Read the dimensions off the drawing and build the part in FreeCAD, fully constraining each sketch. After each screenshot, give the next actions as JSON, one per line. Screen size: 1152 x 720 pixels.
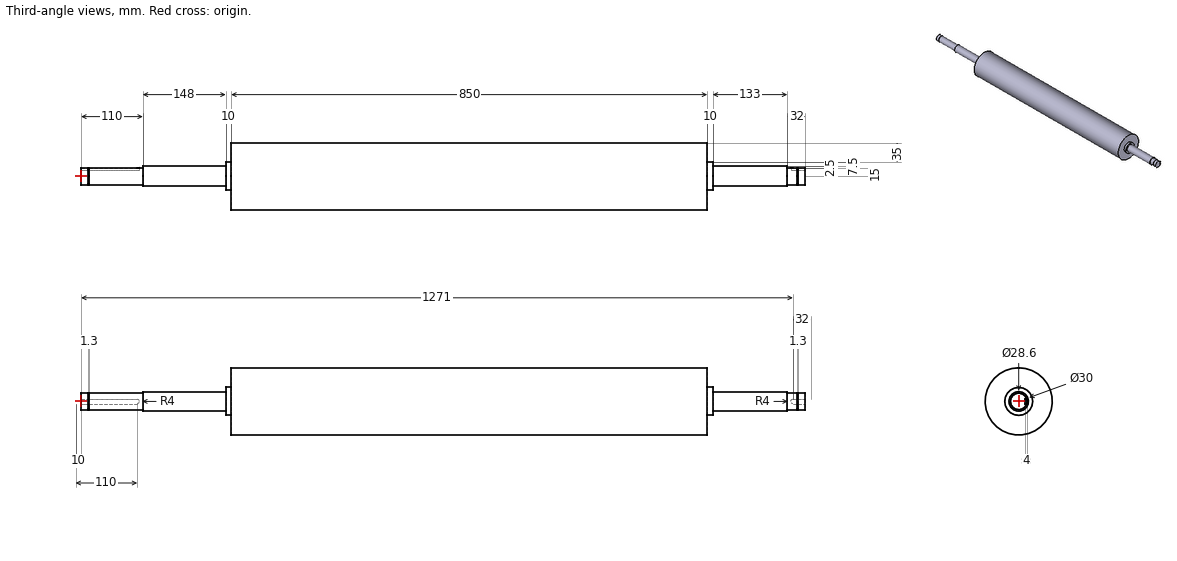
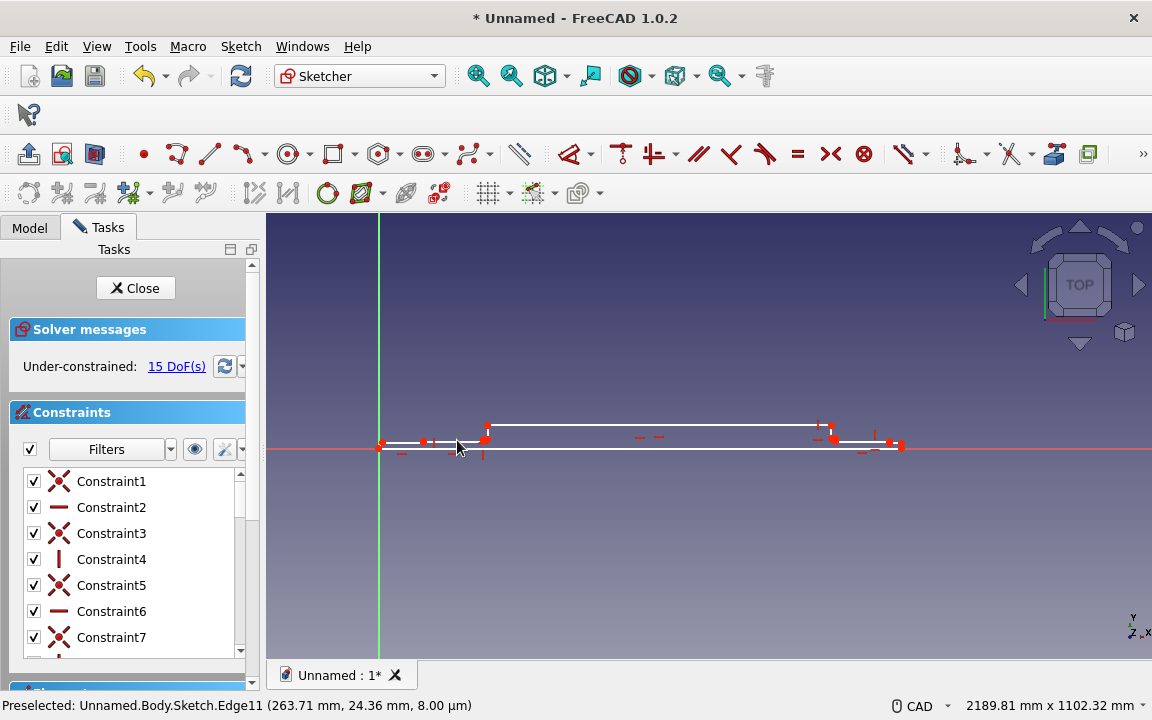
{"action": "scroll", "coordinate": [381, 445], "scroll_direction": "up", "scroll_amount": 10}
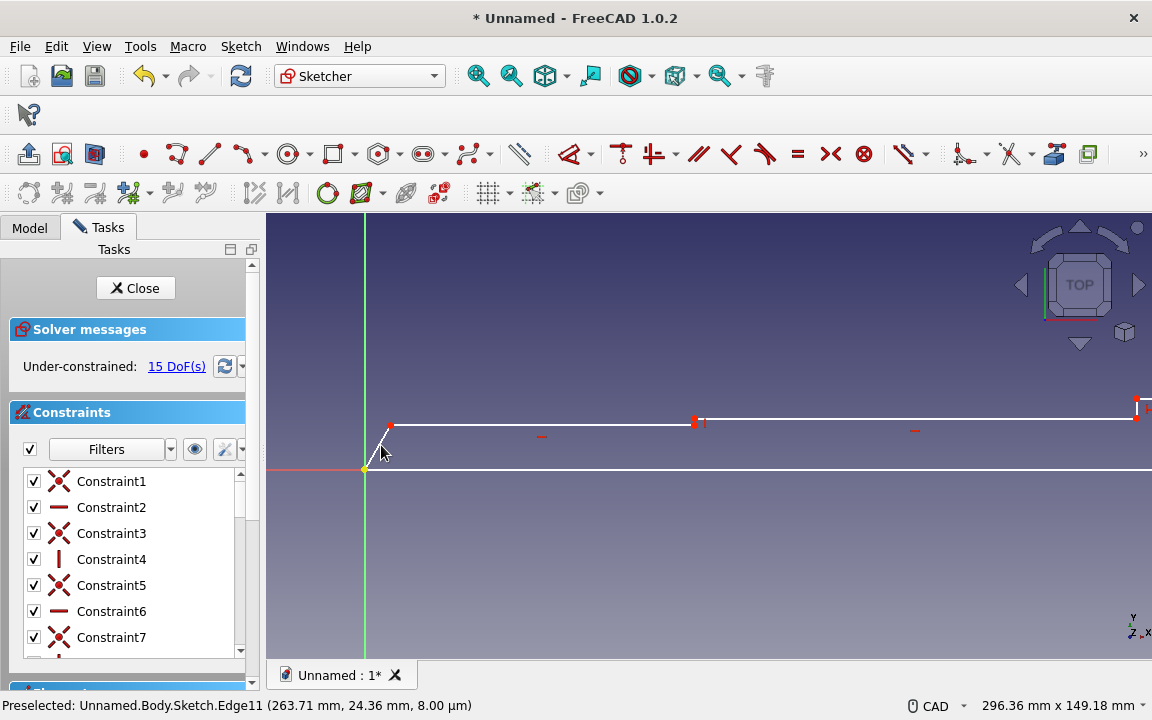
{"action": "left_click", "coordinate": [383, 439]}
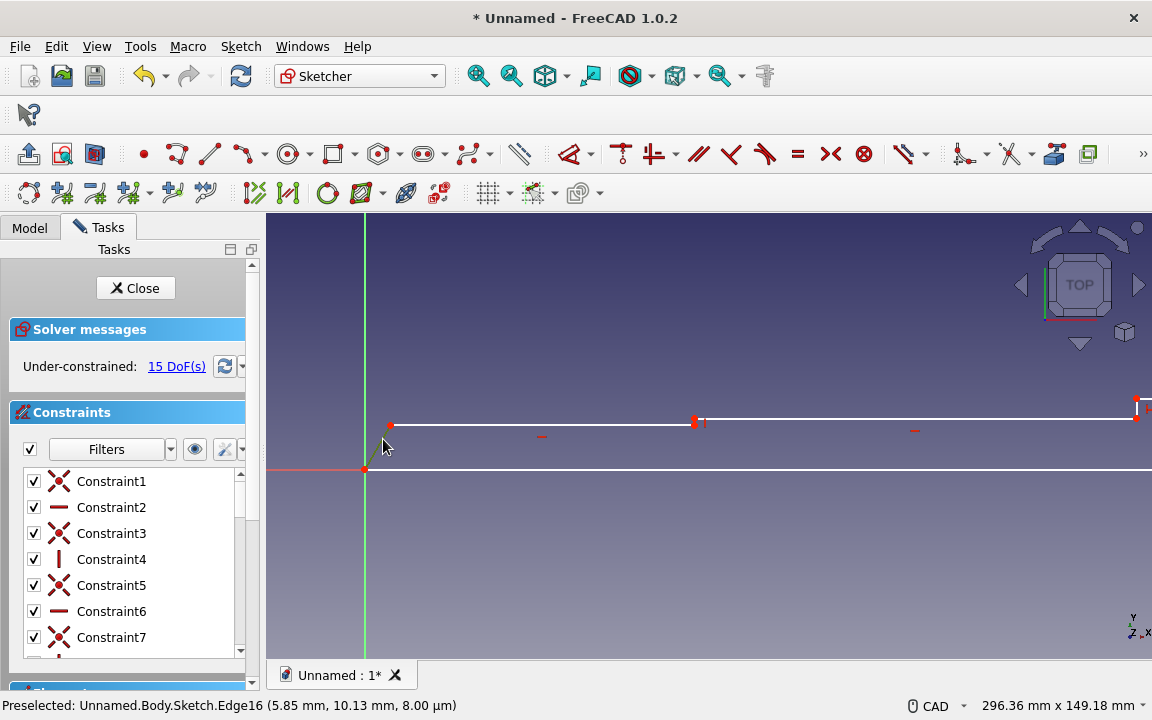
{"action": "left_click", "coordinate": [676, 154]}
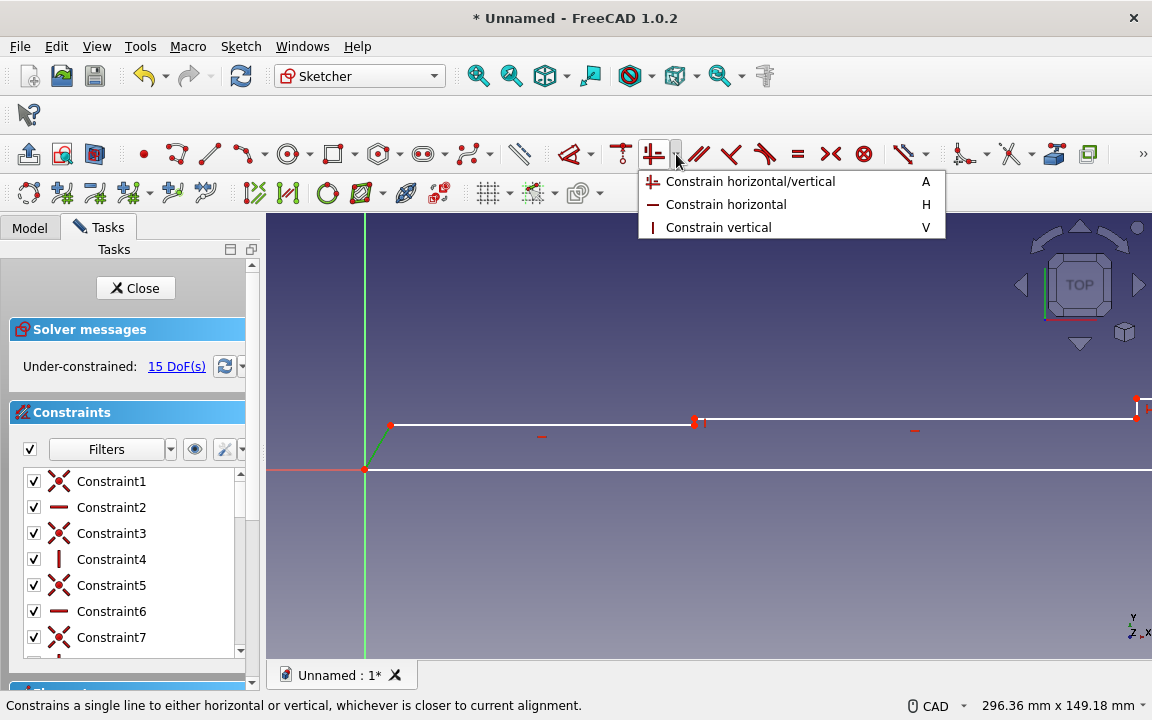
{"action": "left_click", "coordinate": [792, 228]}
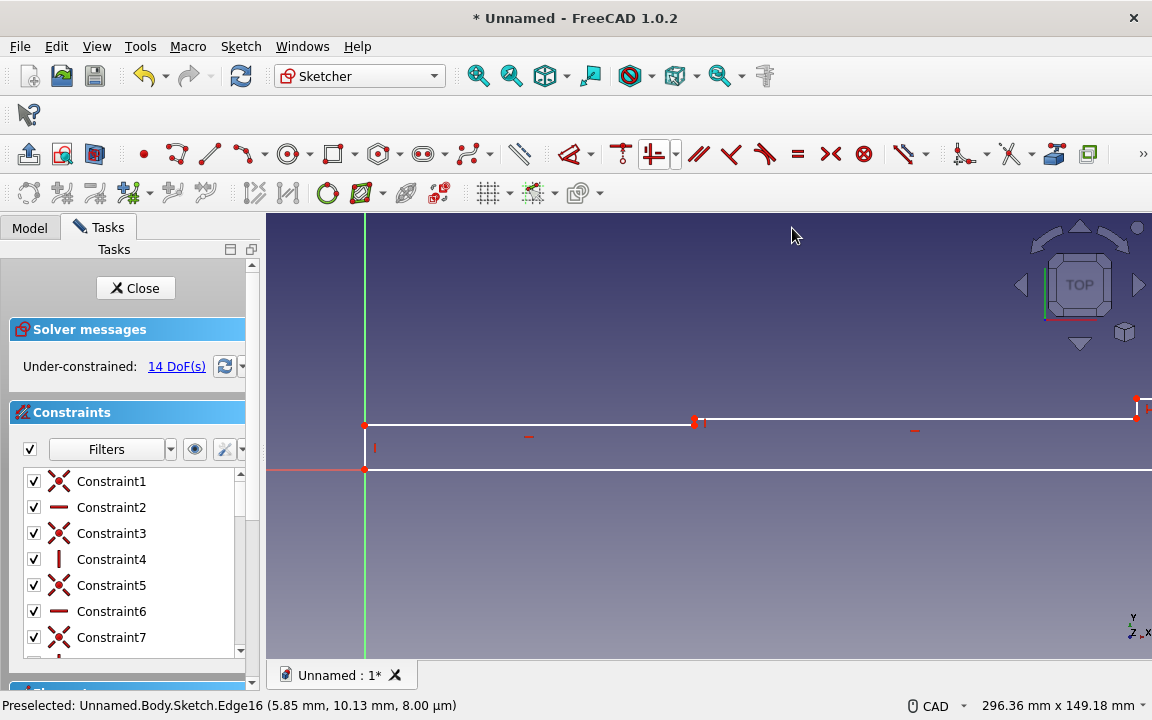
{"action": "key", "text": "d"}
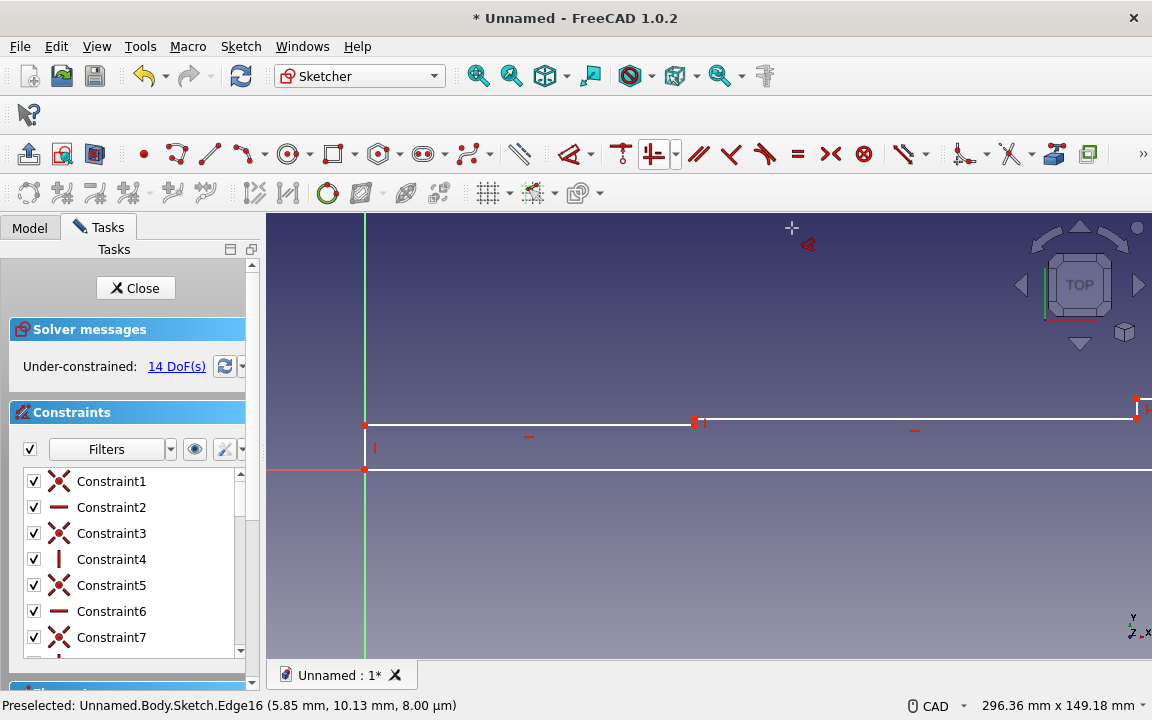
{"action": "scroll", "coordinate": [381, 445], "scroll_direction": "down", "scroll_amount": 10}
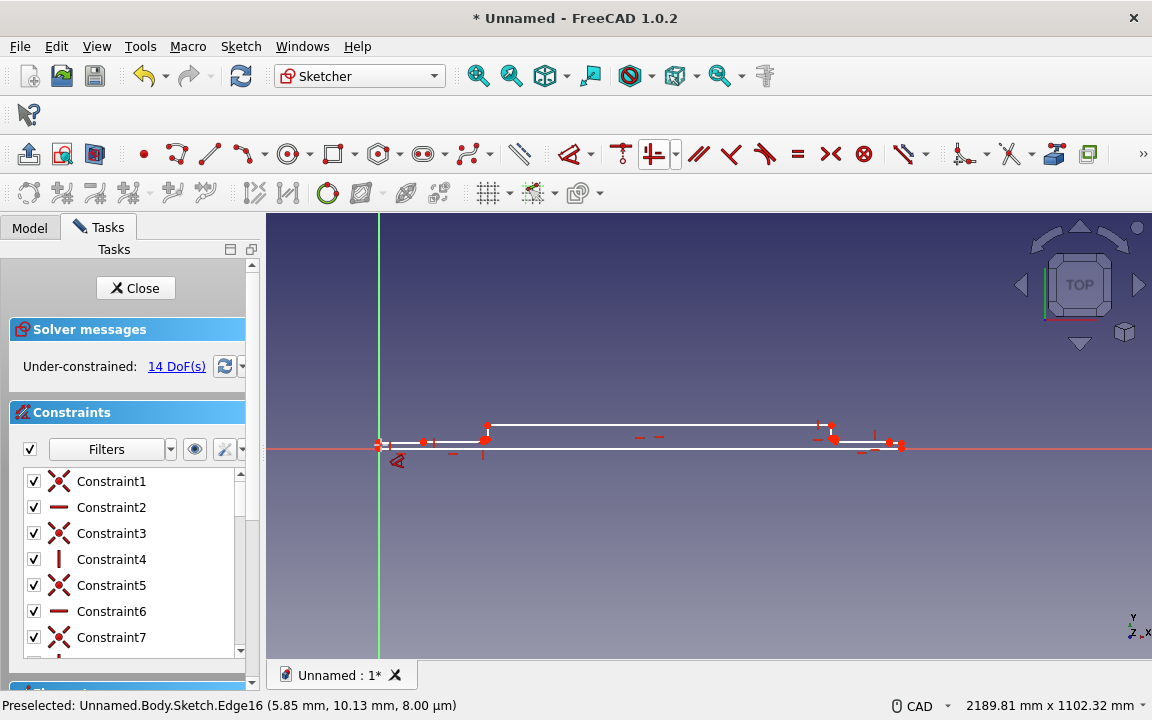
{"action": "scroll", "coordinate": [902, 447], "scroll_direction": "up", "scroll_amount": 11}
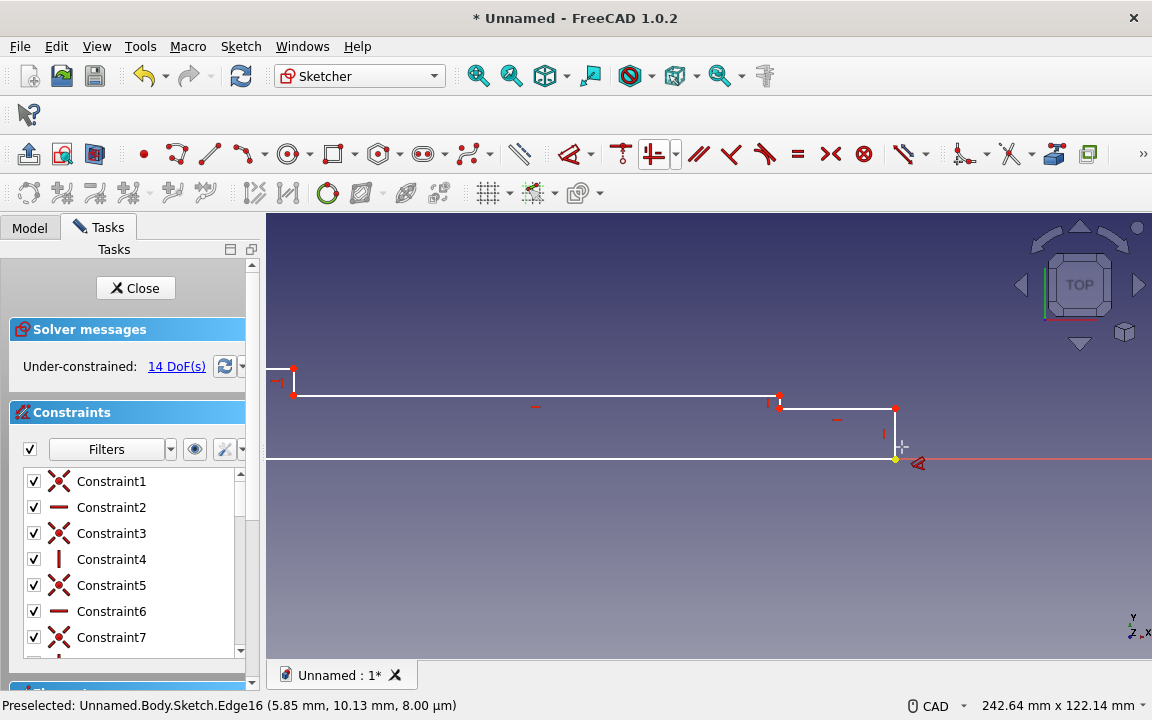
{"action": "left_click", "coordinate": [895, 444]}
{"action": "left_click", "coordinate": [929, 434]}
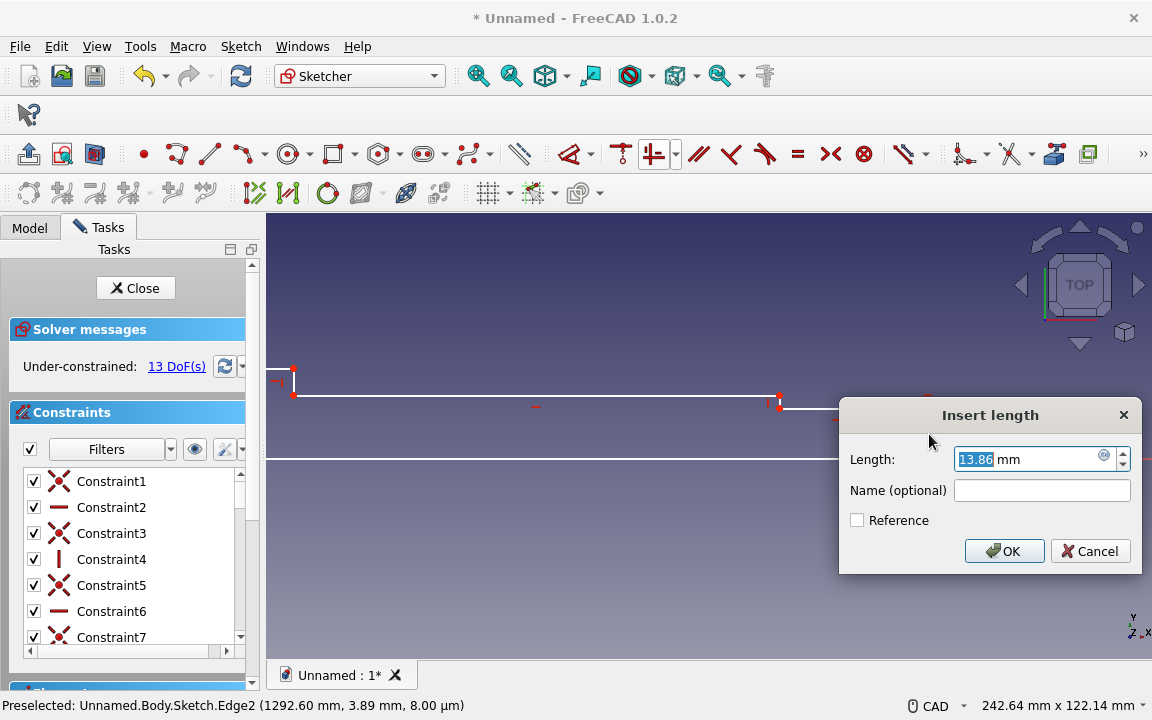
{"action": "type", "text": "15"}
{"action": "key", "text": "Return"}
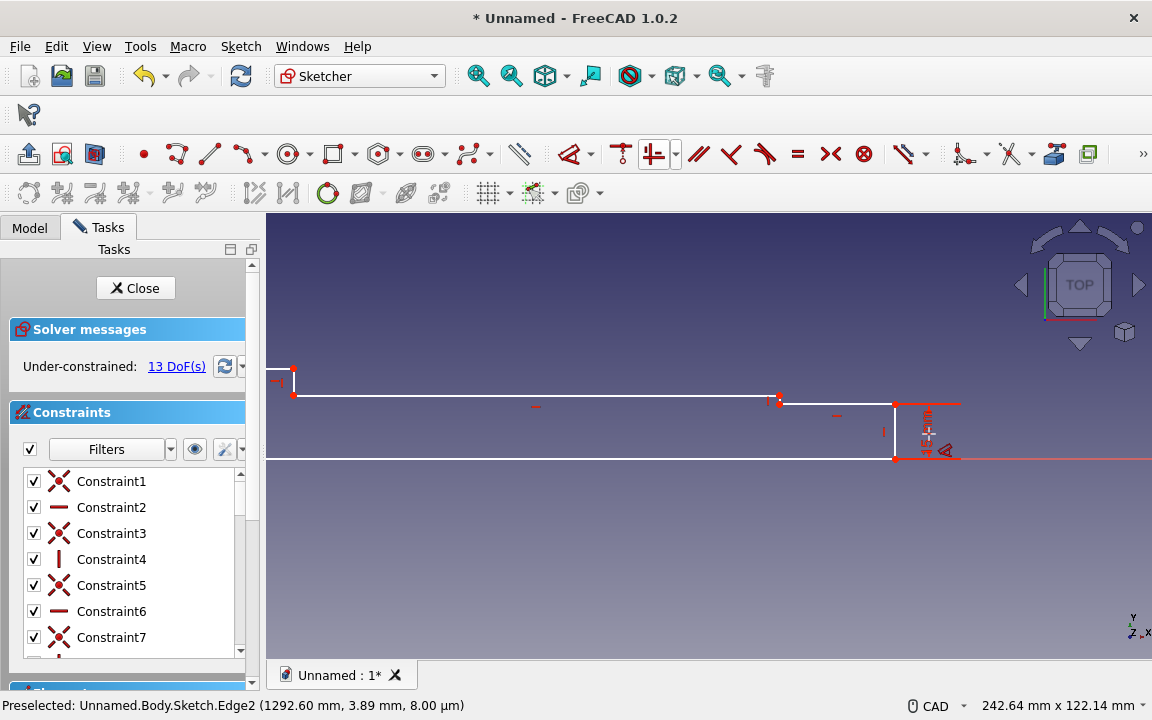
{"action": "left_click", "coordinate": [861, 404]}
{"action": "left_click", "coordinate": [838, 438]}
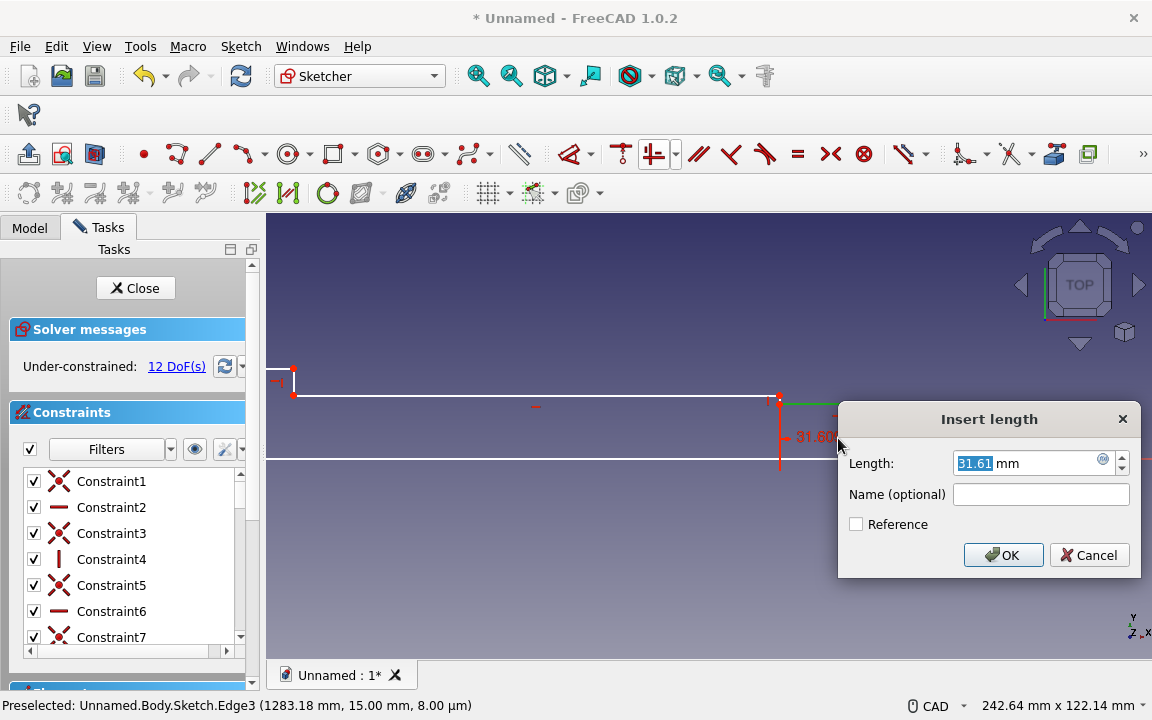
{"action": "type", "text": "32"}
{"action": "key", "text": "Return"}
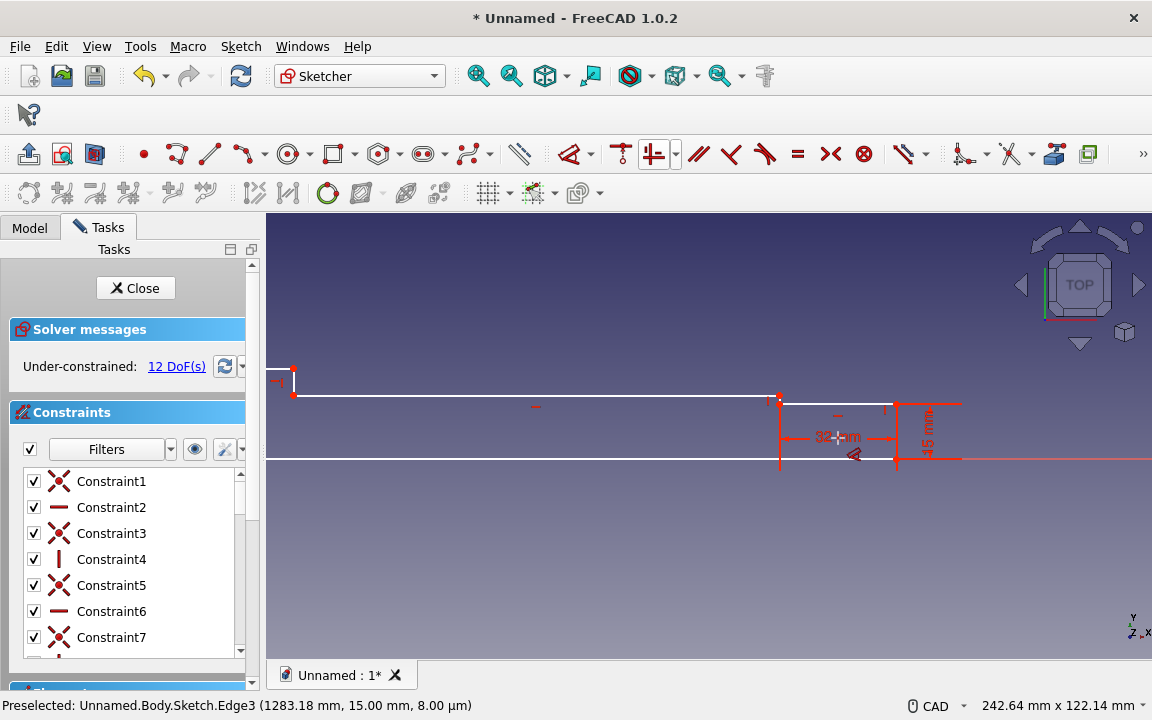
{"action": "scroll", "coordinate": [903, 447], "scroll_direction": "down", "scroll_amount": 11}